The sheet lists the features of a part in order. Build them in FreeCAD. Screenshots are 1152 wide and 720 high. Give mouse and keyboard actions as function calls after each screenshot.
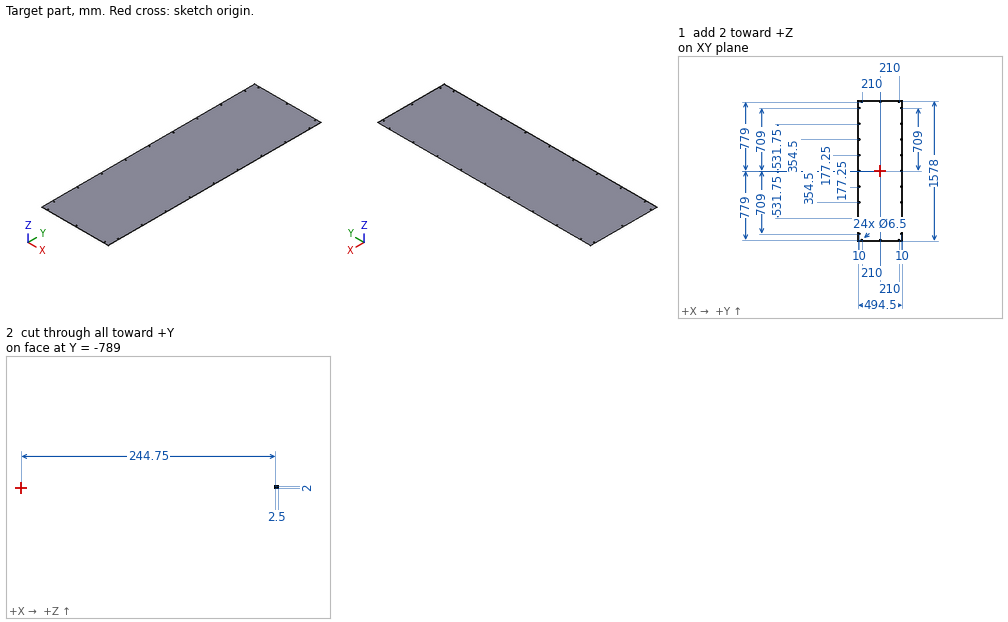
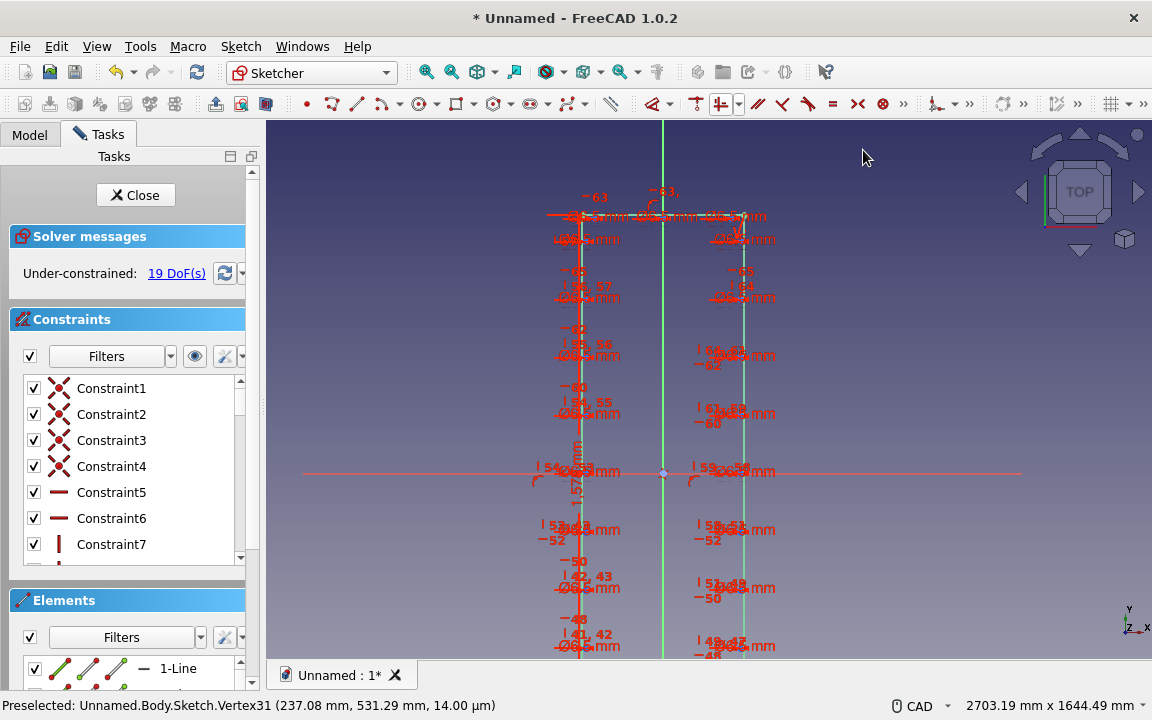
click(663, 219)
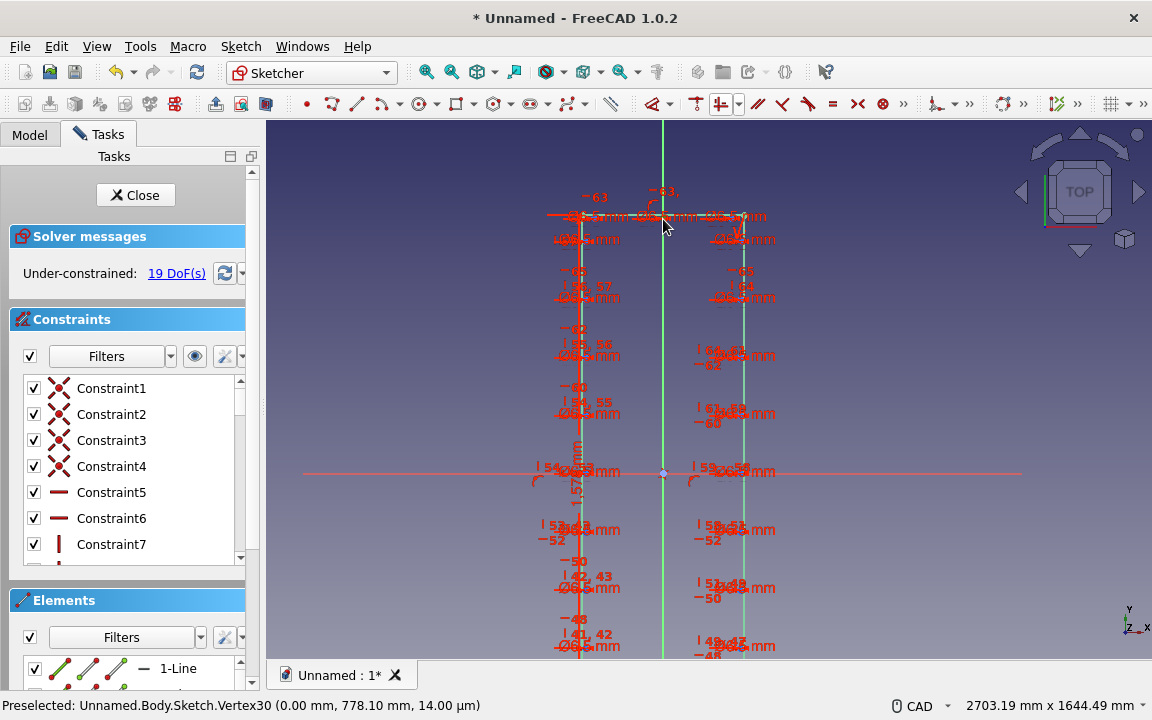
click(732, 219)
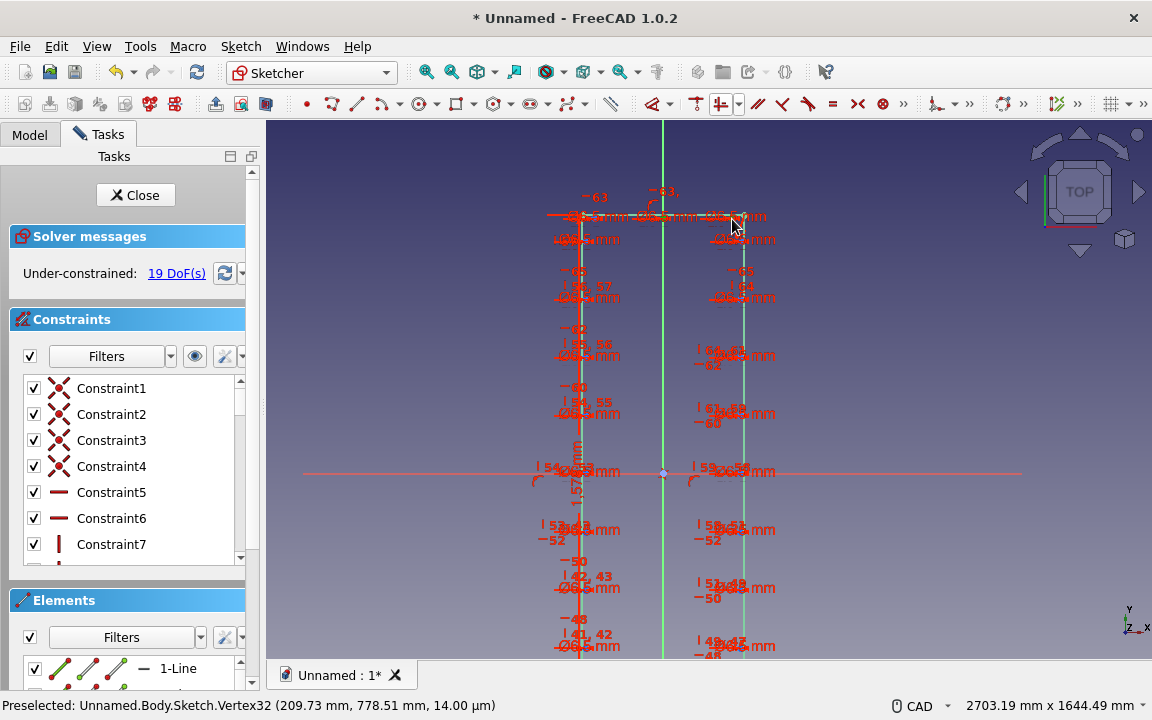
click(738, 104)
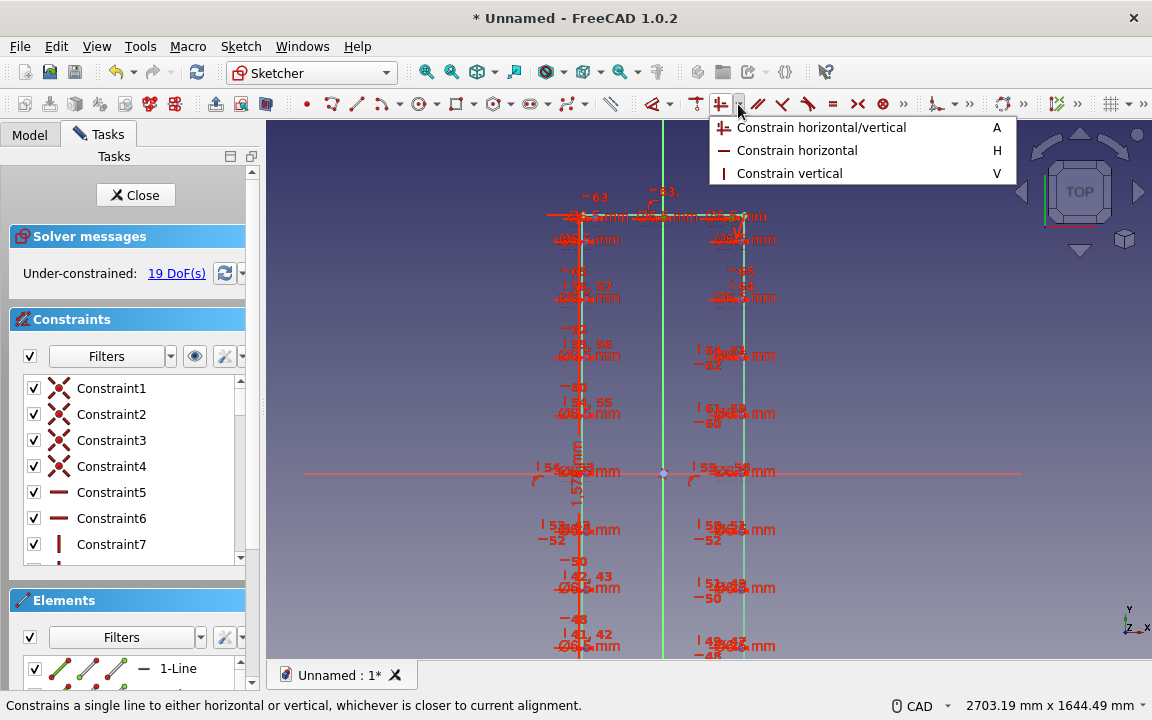
click(863, 150)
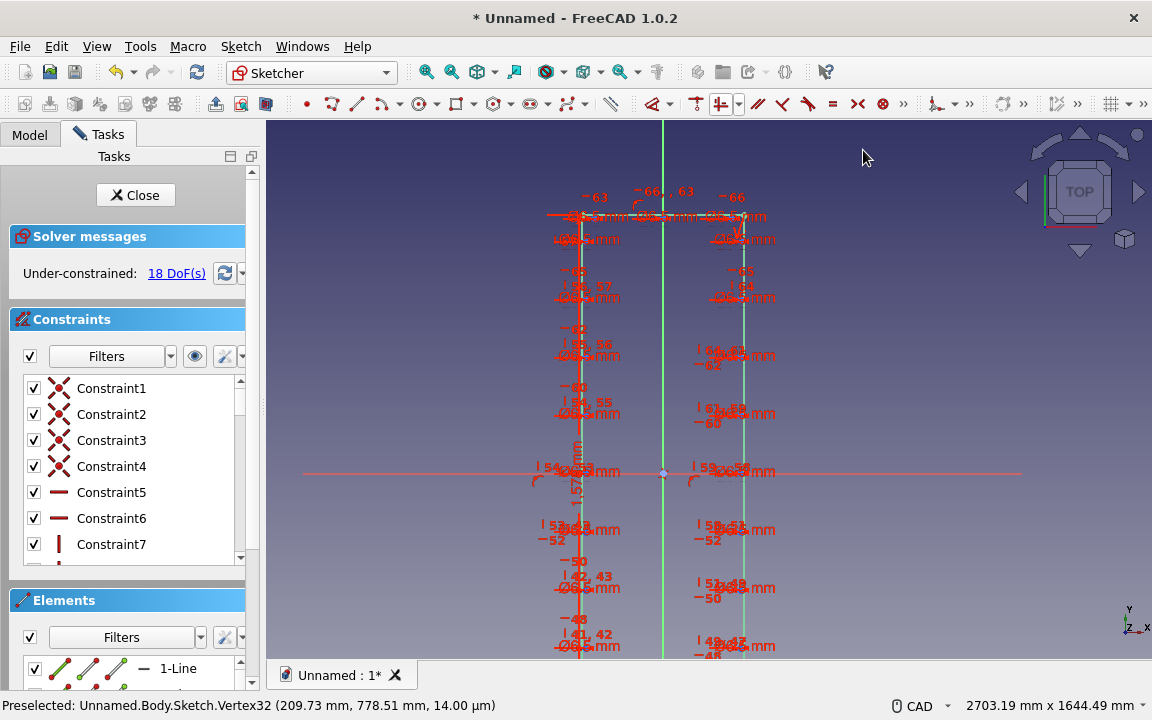
click(741, 300)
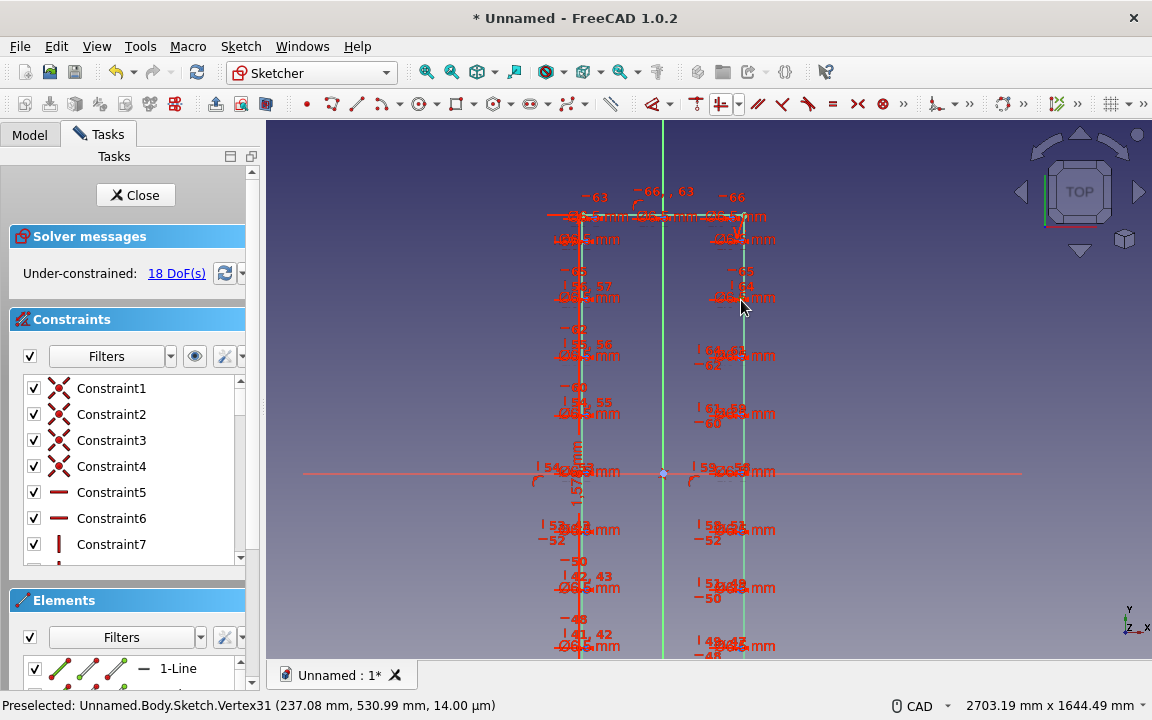
click(741, 242)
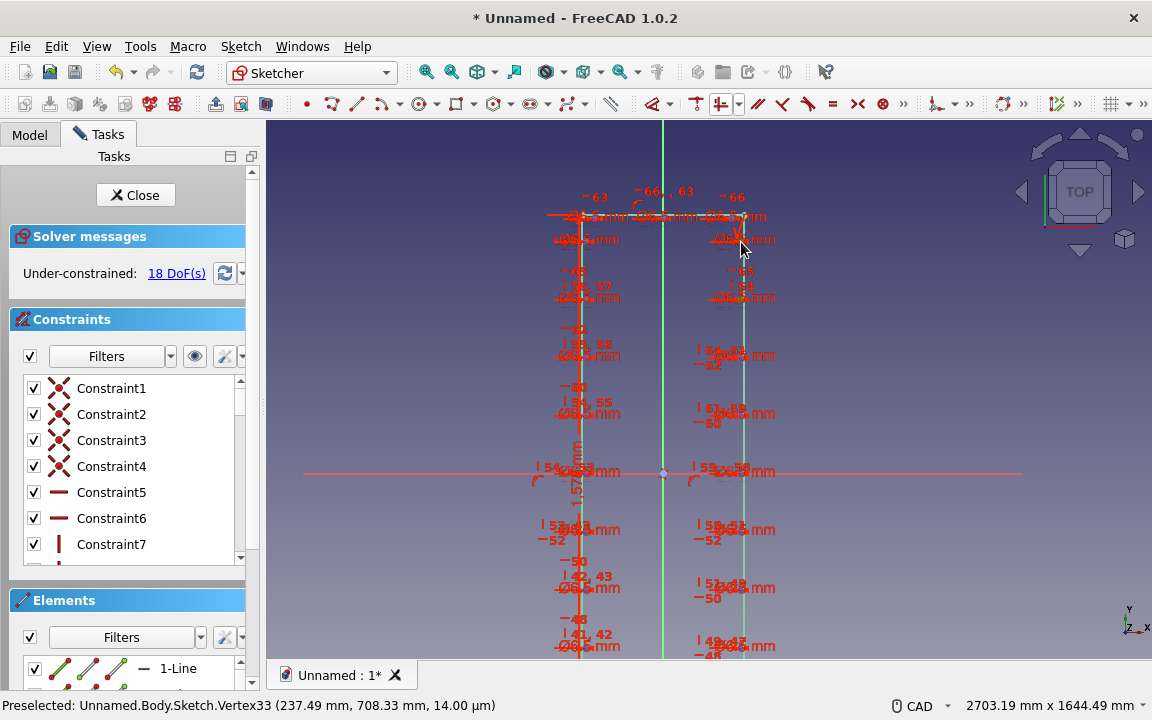
key(v)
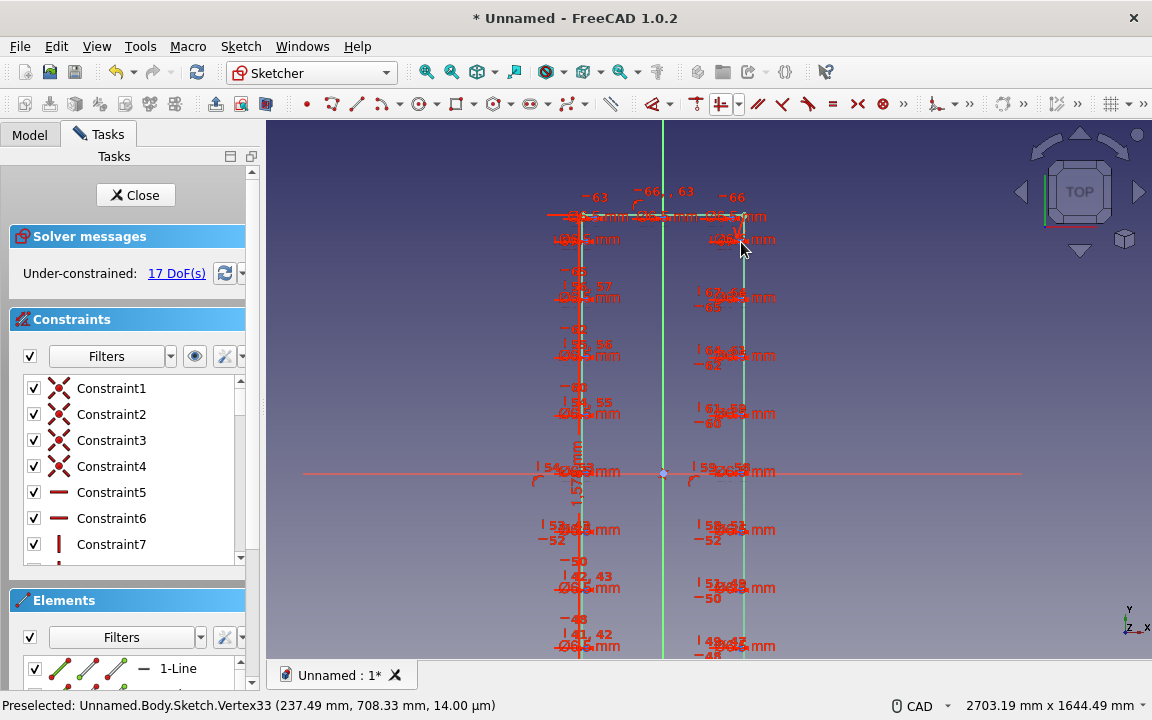
click(652, 104)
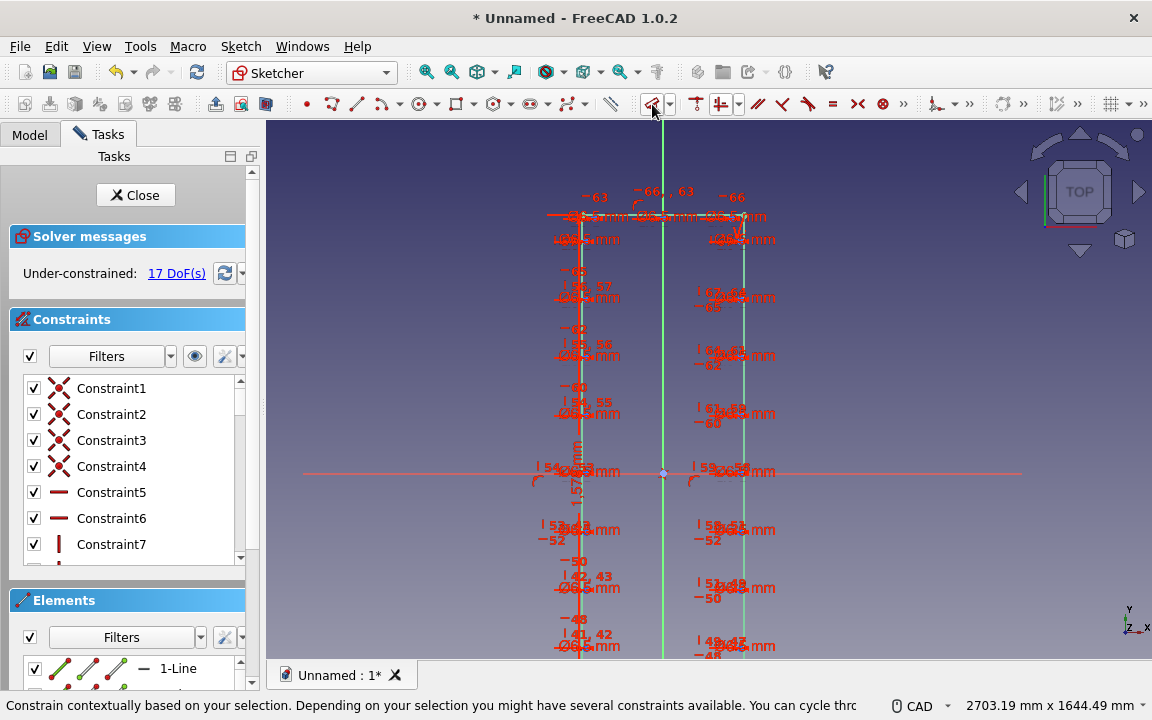
scroll(594, 218, down, 2)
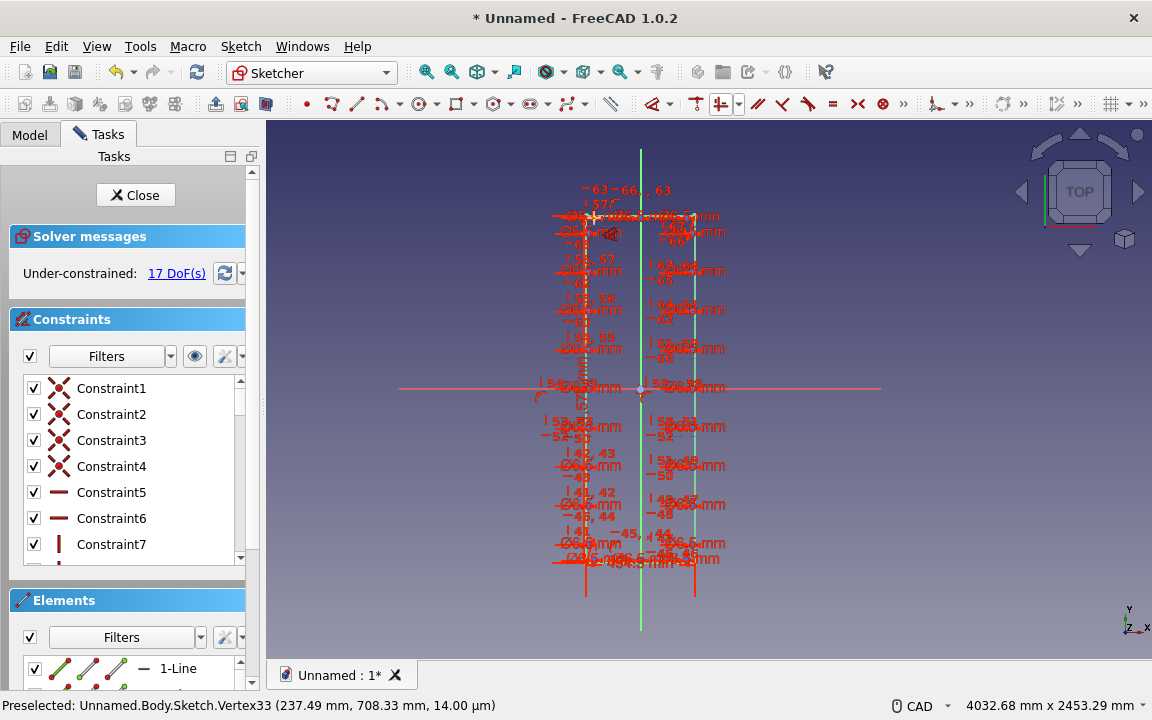
click(588, 545)
click(554, 467)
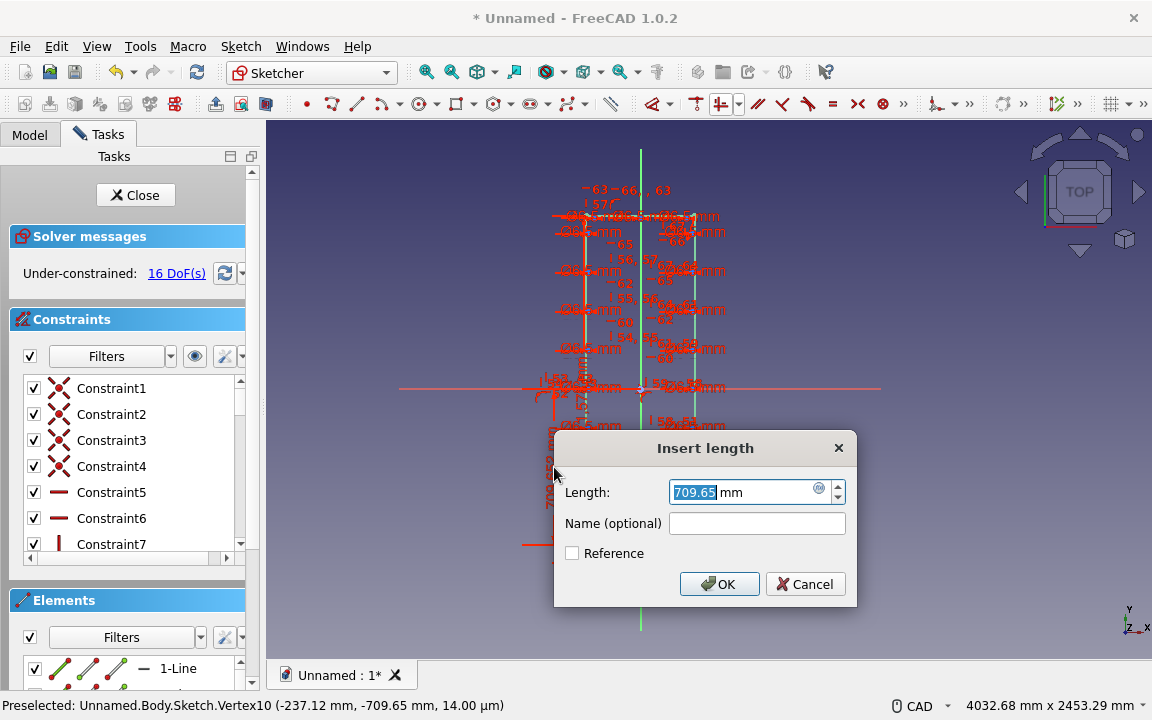
text(709)
key(Return)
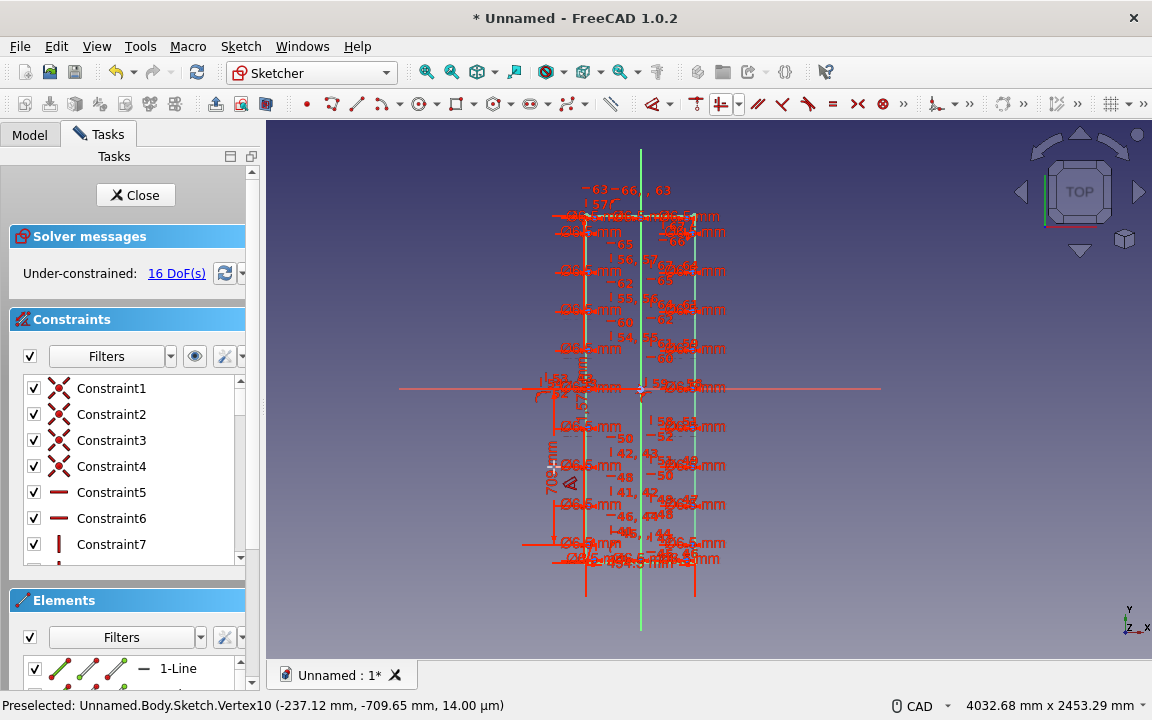
scroll(594, 561, up, 2)